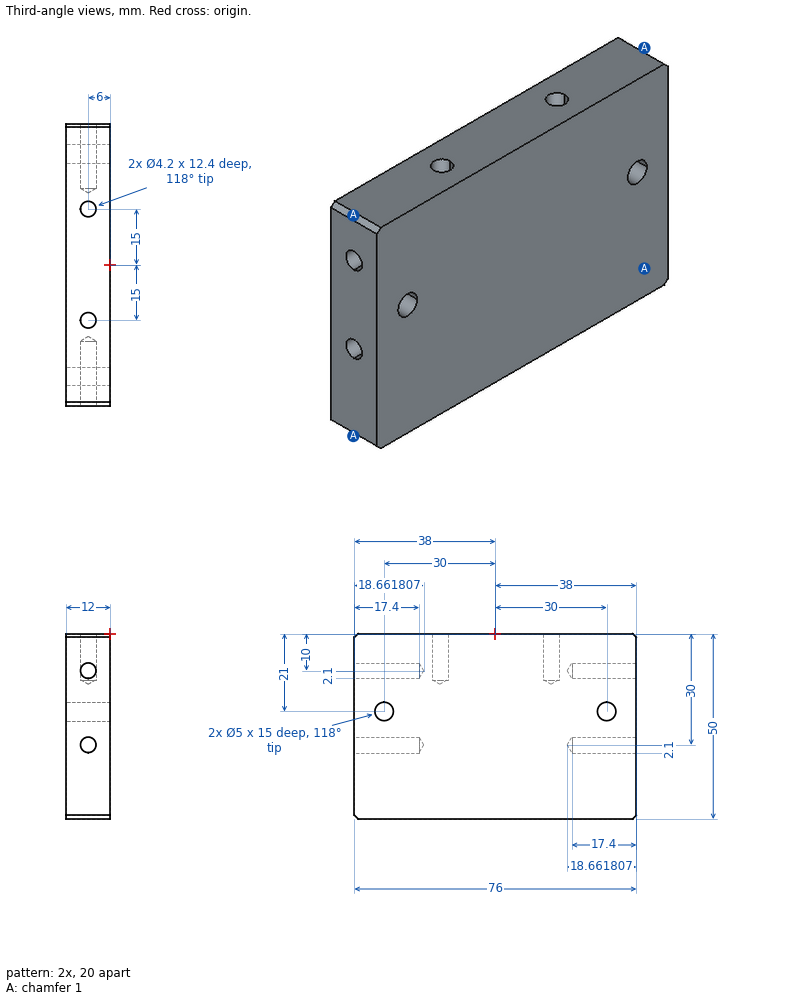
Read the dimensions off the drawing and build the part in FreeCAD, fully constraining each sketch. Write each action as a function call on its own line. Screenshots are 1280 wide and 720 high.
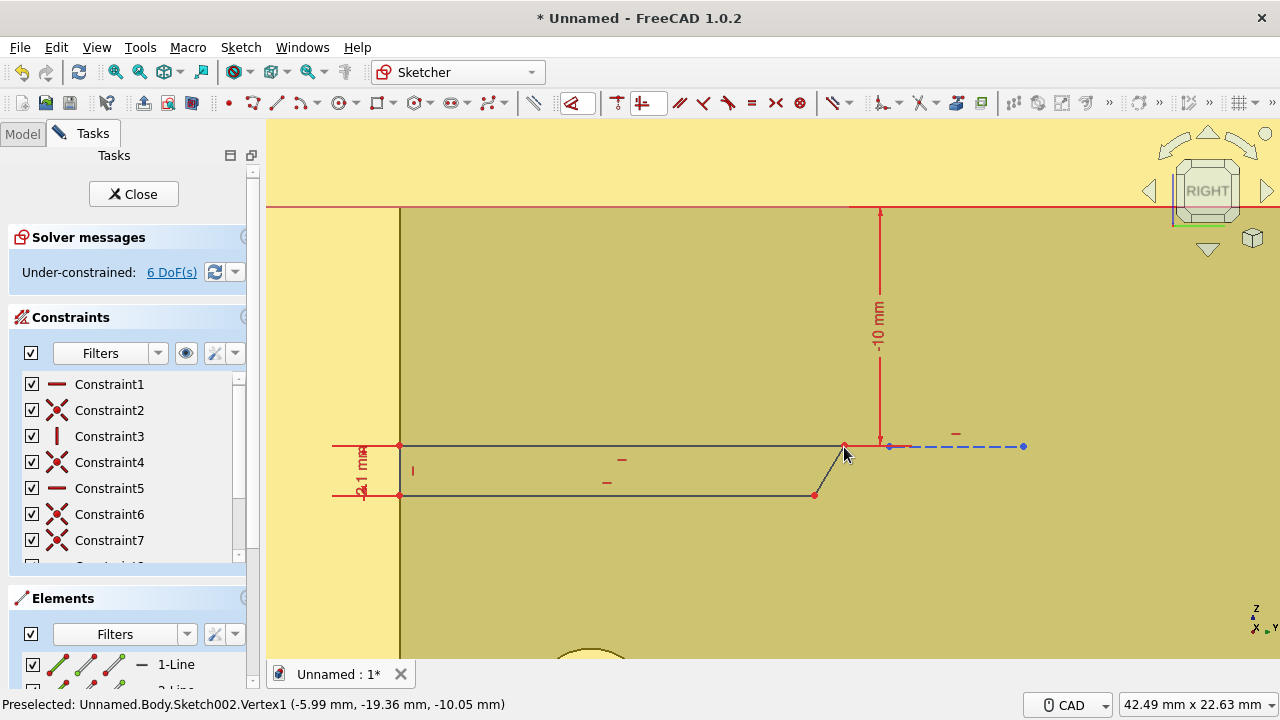
click(400, 446)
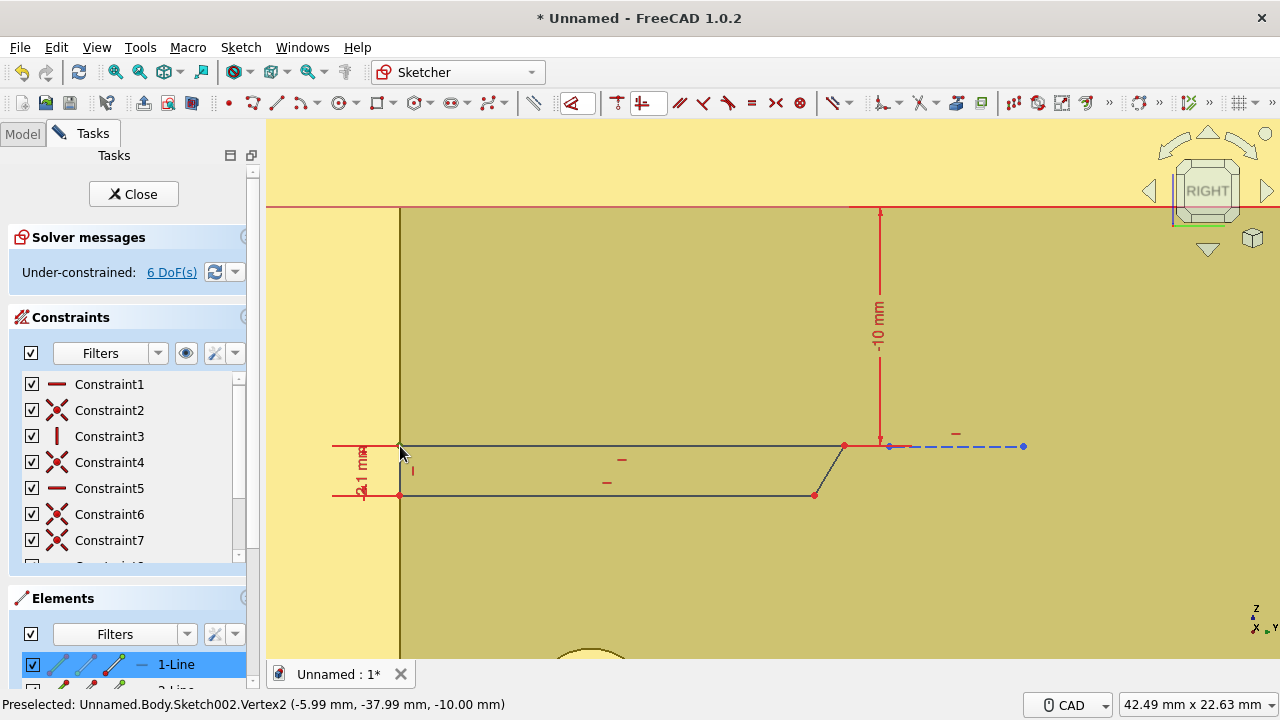
key(l)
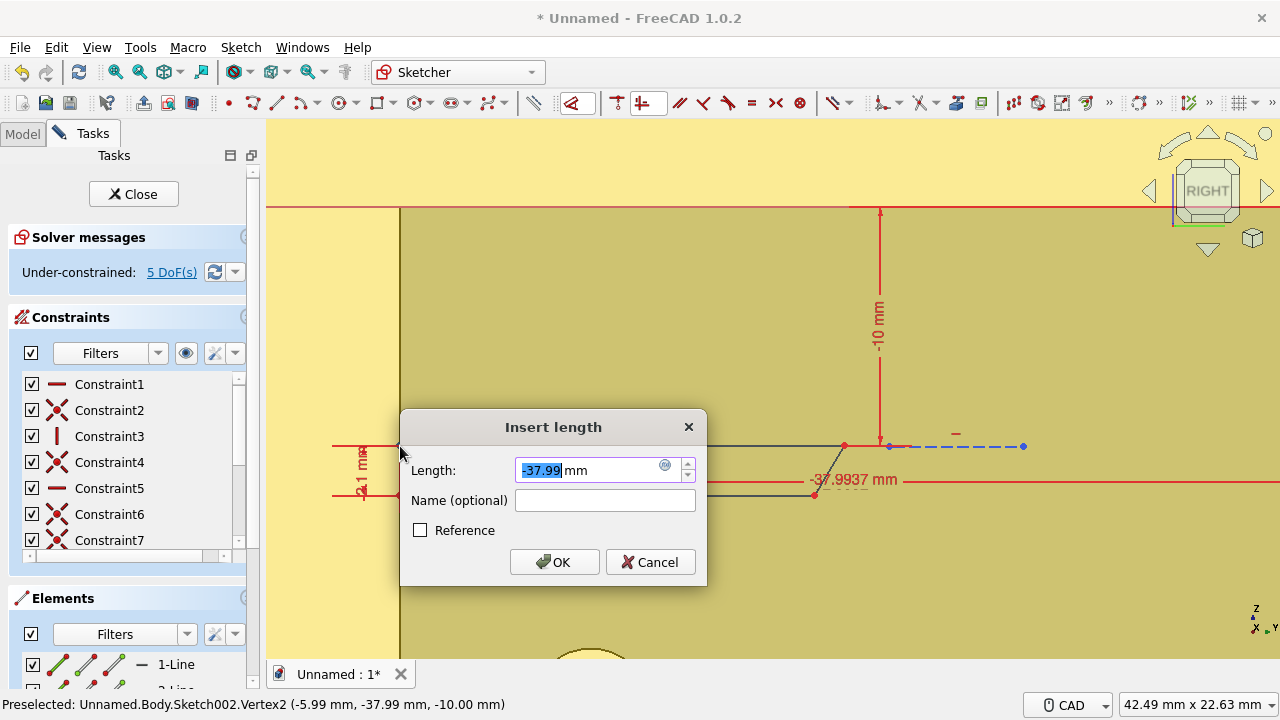
text(-38)
key(Return)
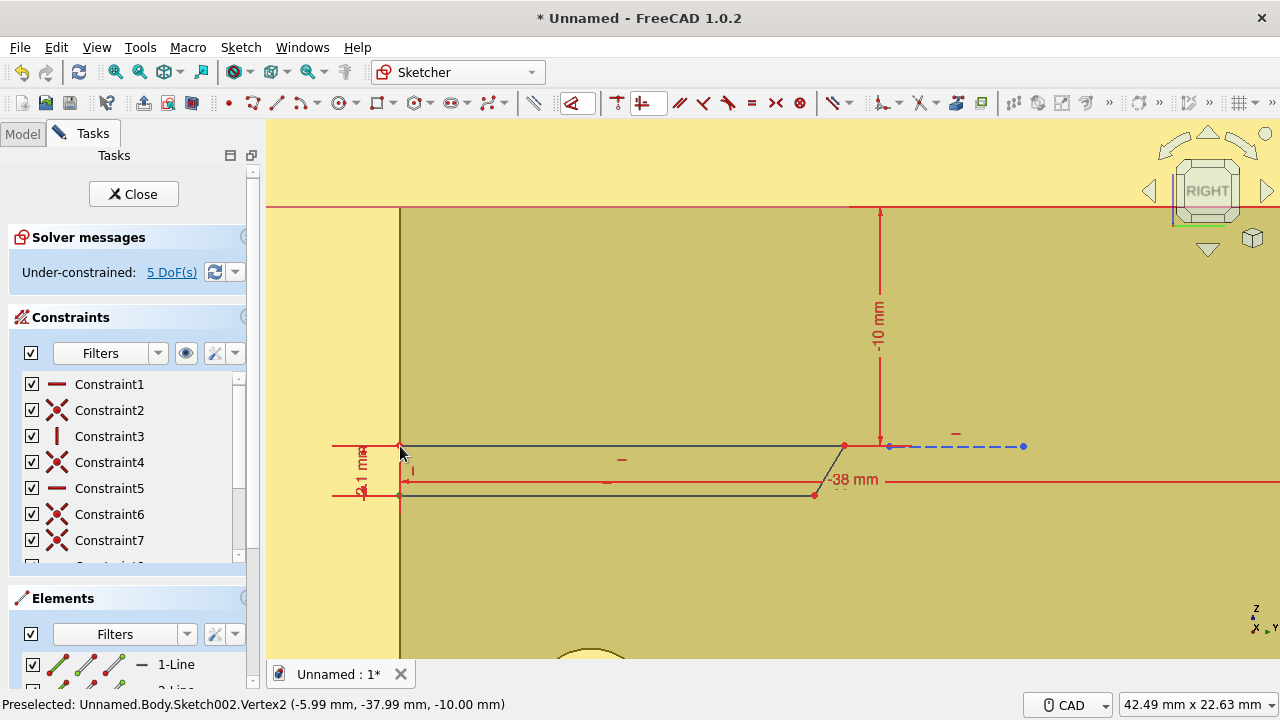
click(889, 447)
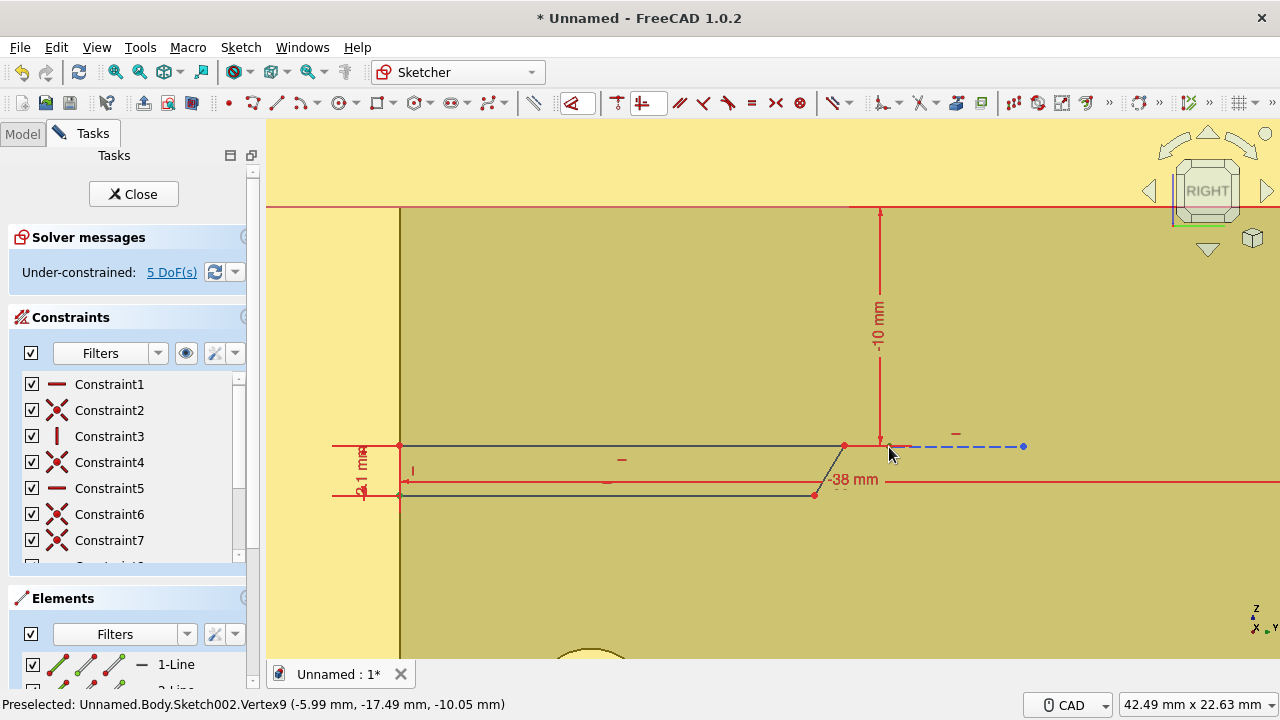
key(i)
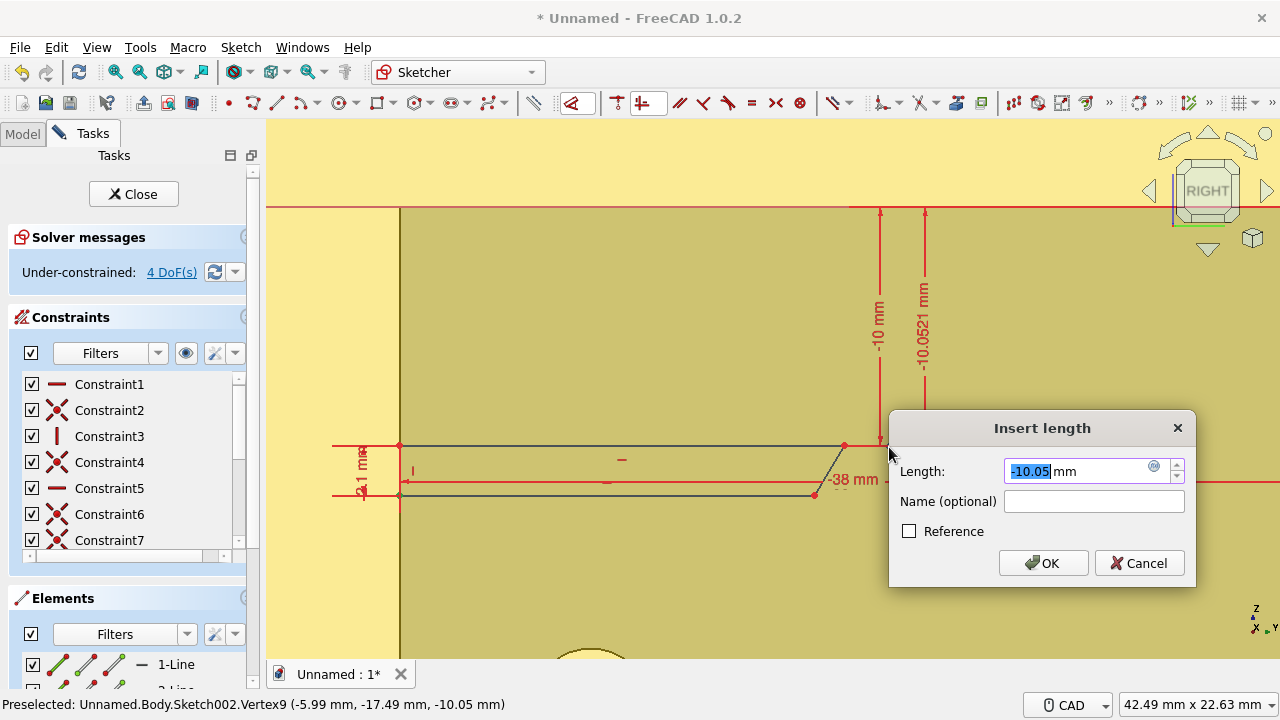
text(-10)
key(Return)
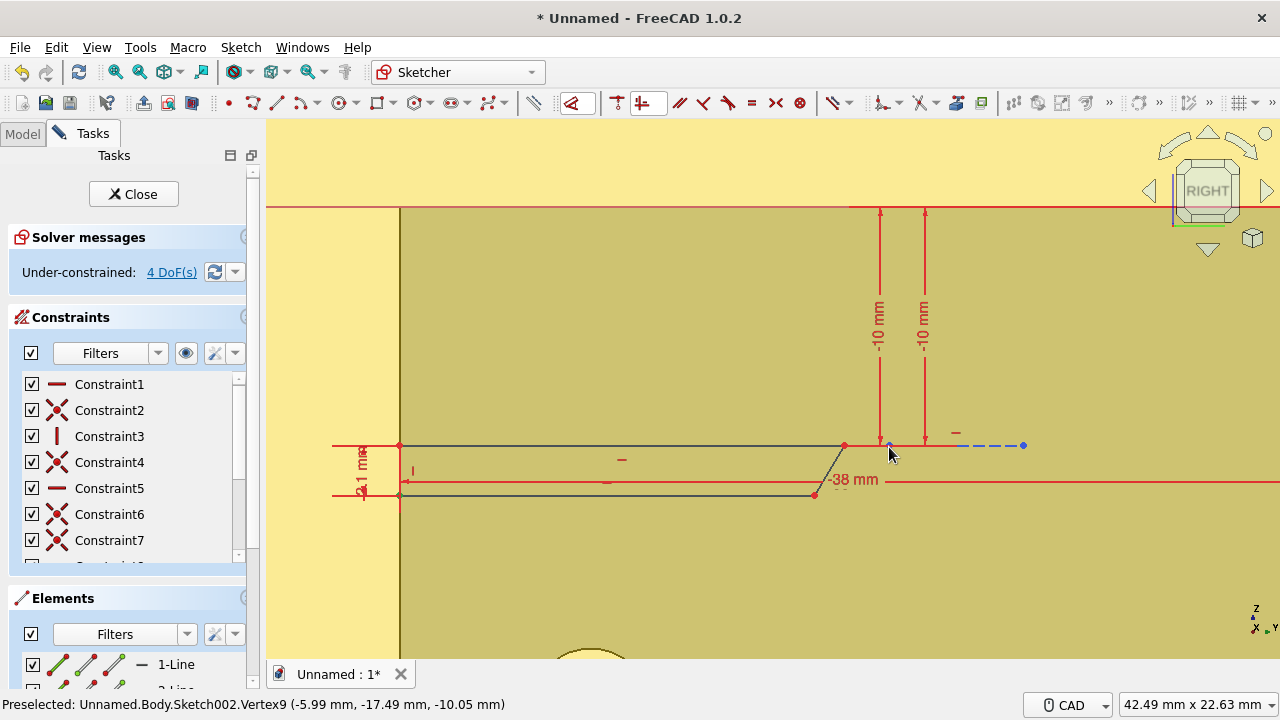
click(524, 496)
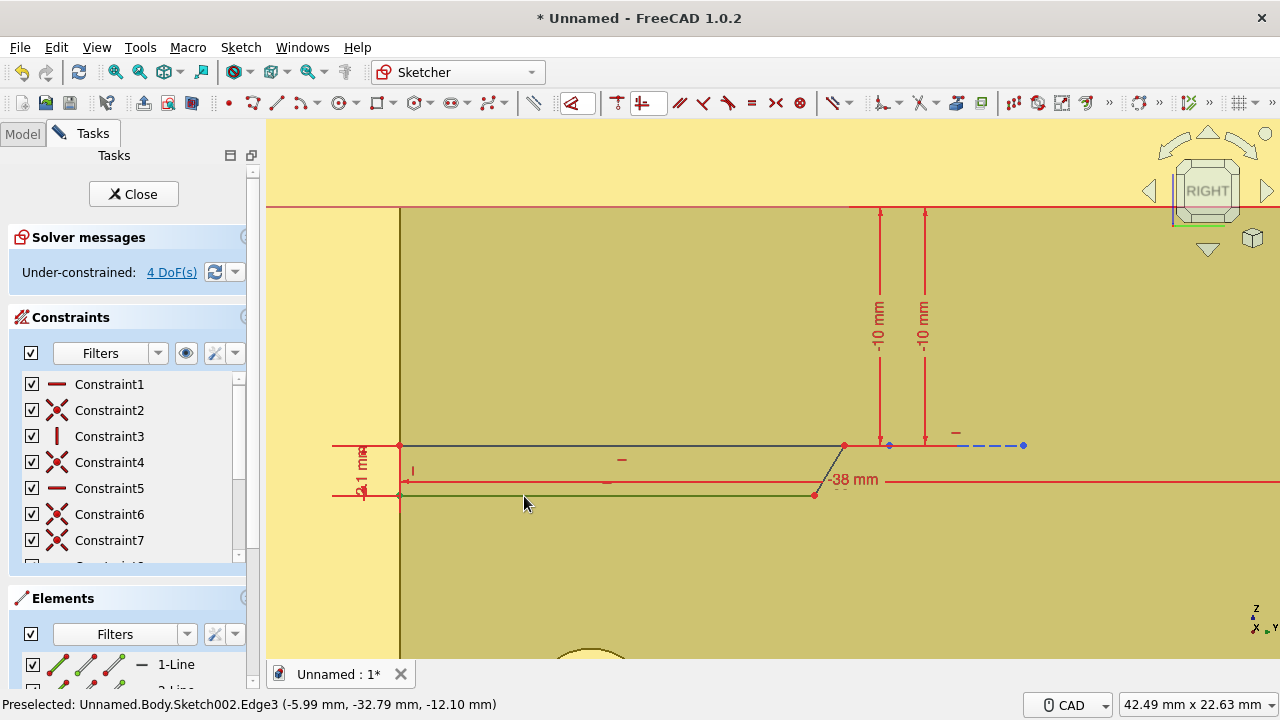
key(l)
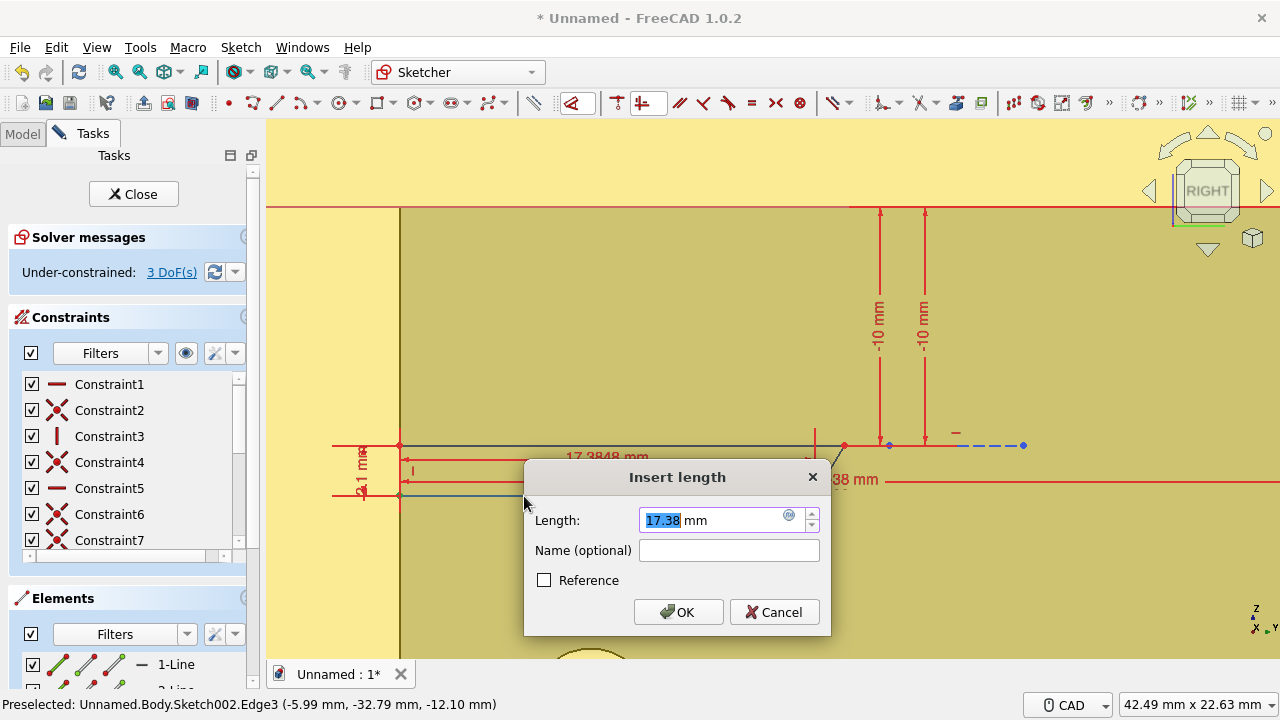
text(17.4)
key(Return)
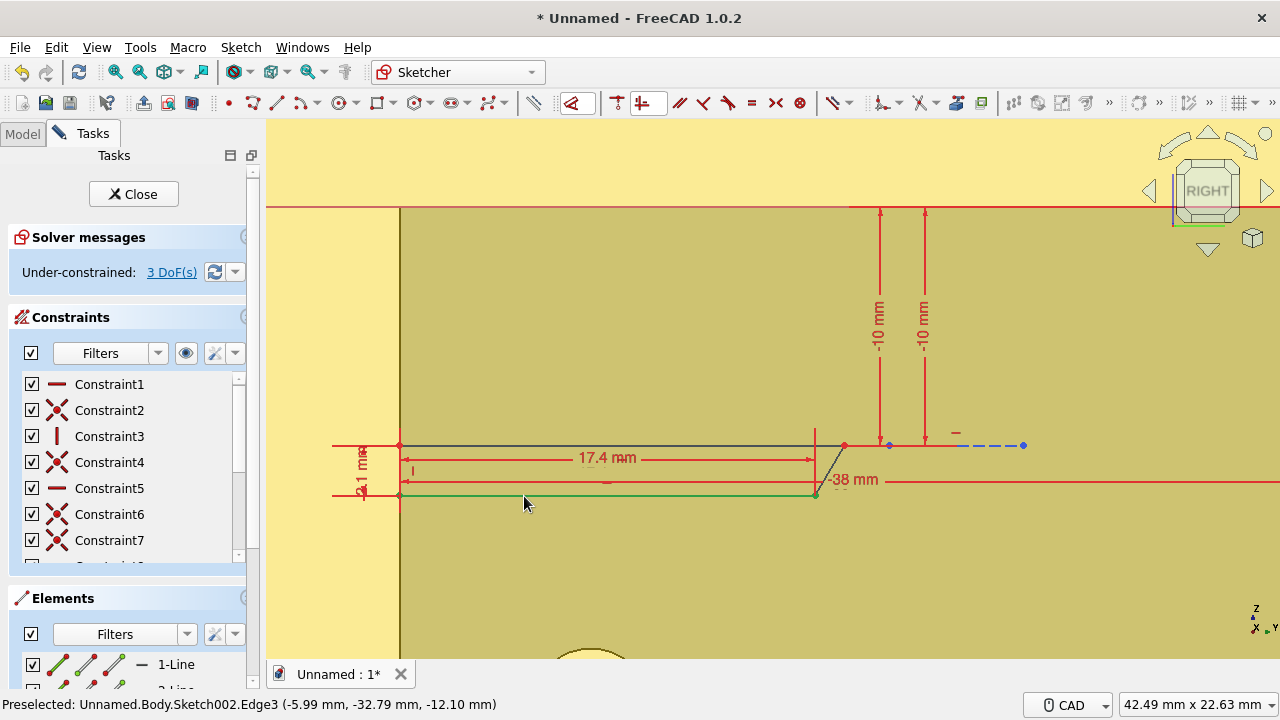
click(711, 446)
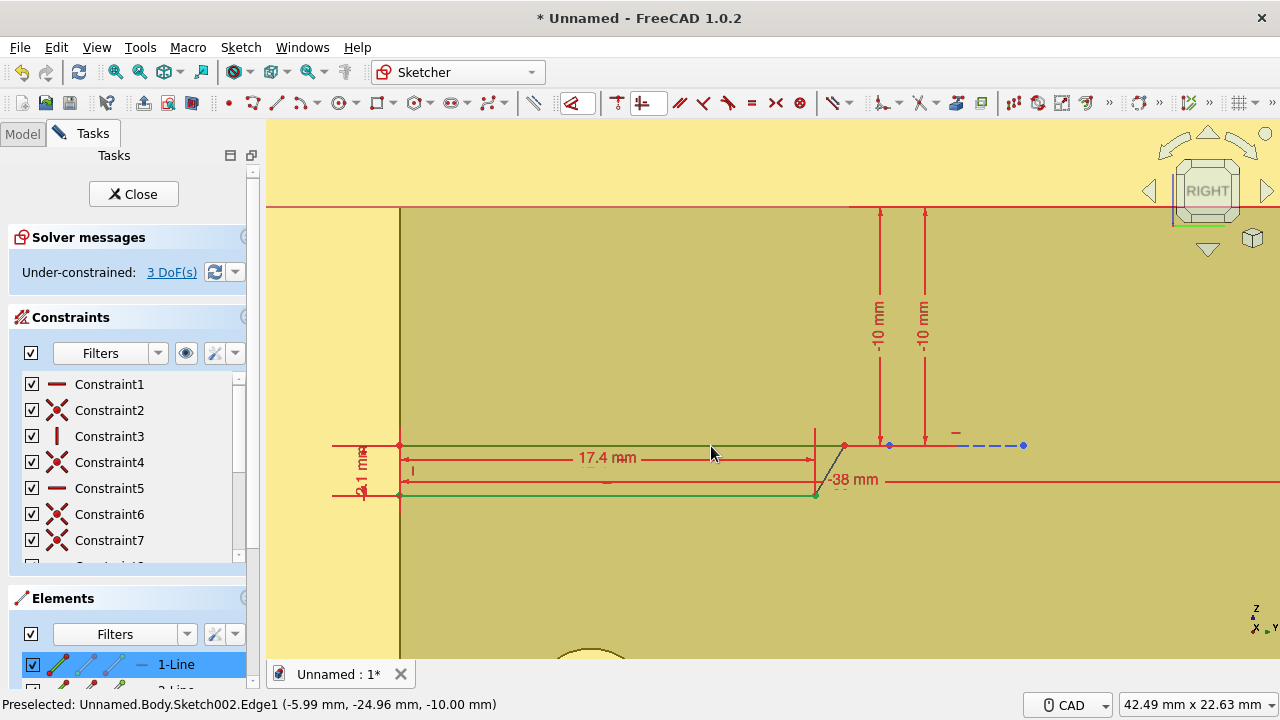
click(590, 104)